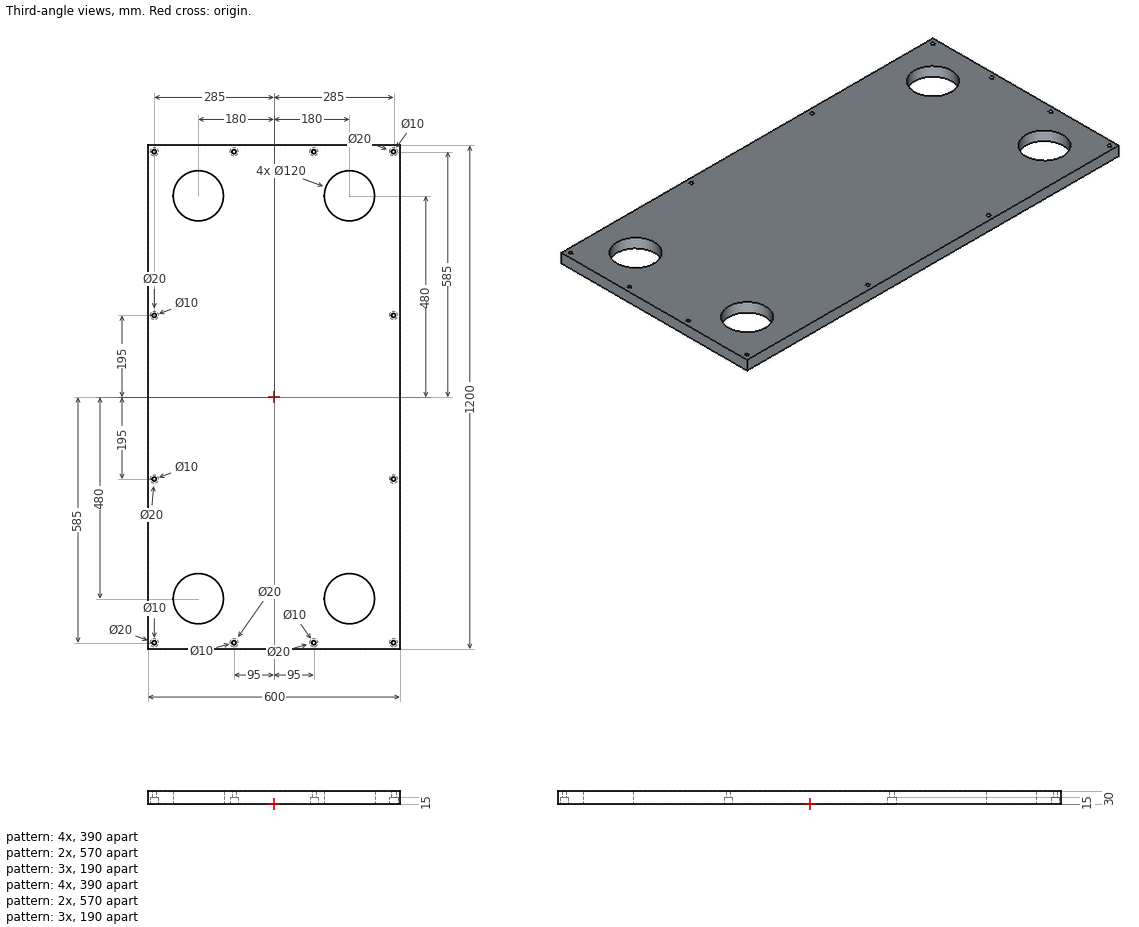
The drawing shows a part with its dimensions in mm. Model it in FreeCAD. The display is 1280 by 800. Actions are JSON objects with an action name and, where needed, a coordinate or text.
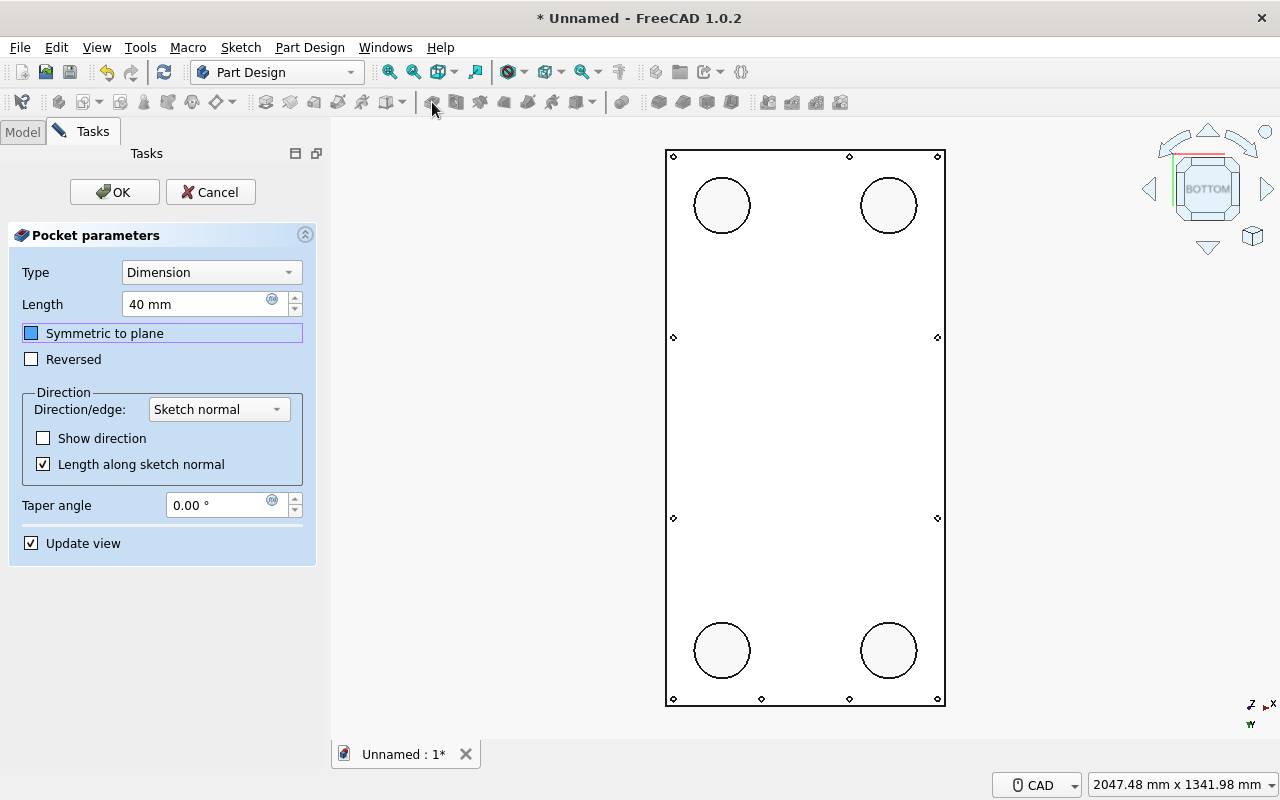
{"action": "left_click", "coordinate": [115, 192]}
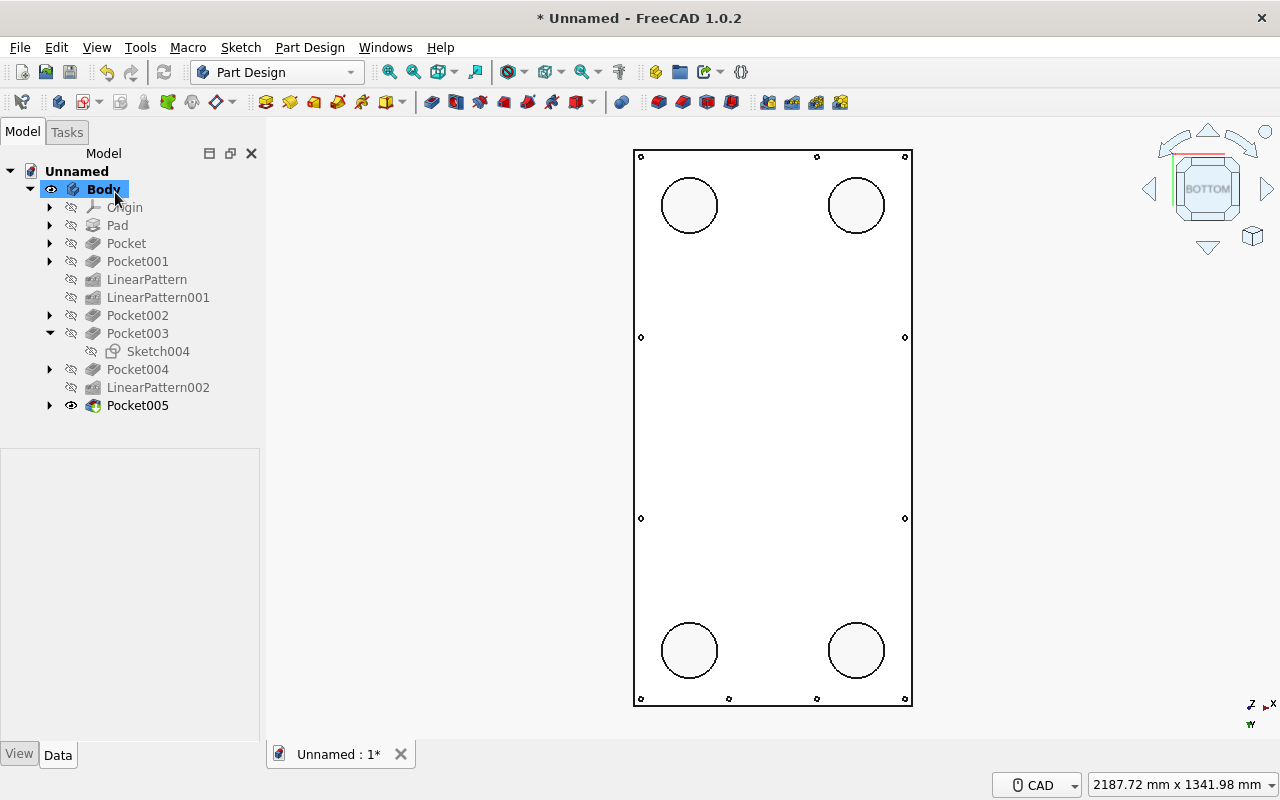
{"action": "left_click", "coordinate": [84, 102]}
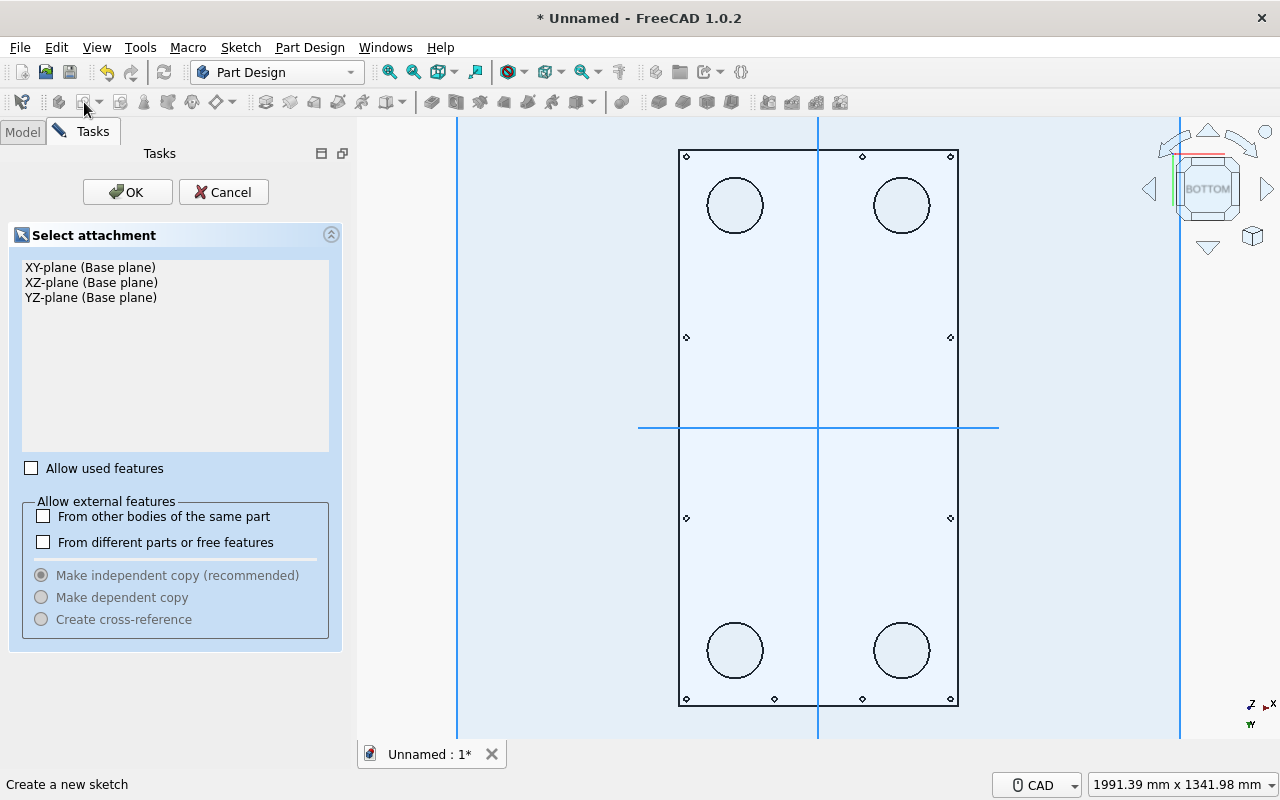
{"action": "left_click", "coordinate": [82, 268]}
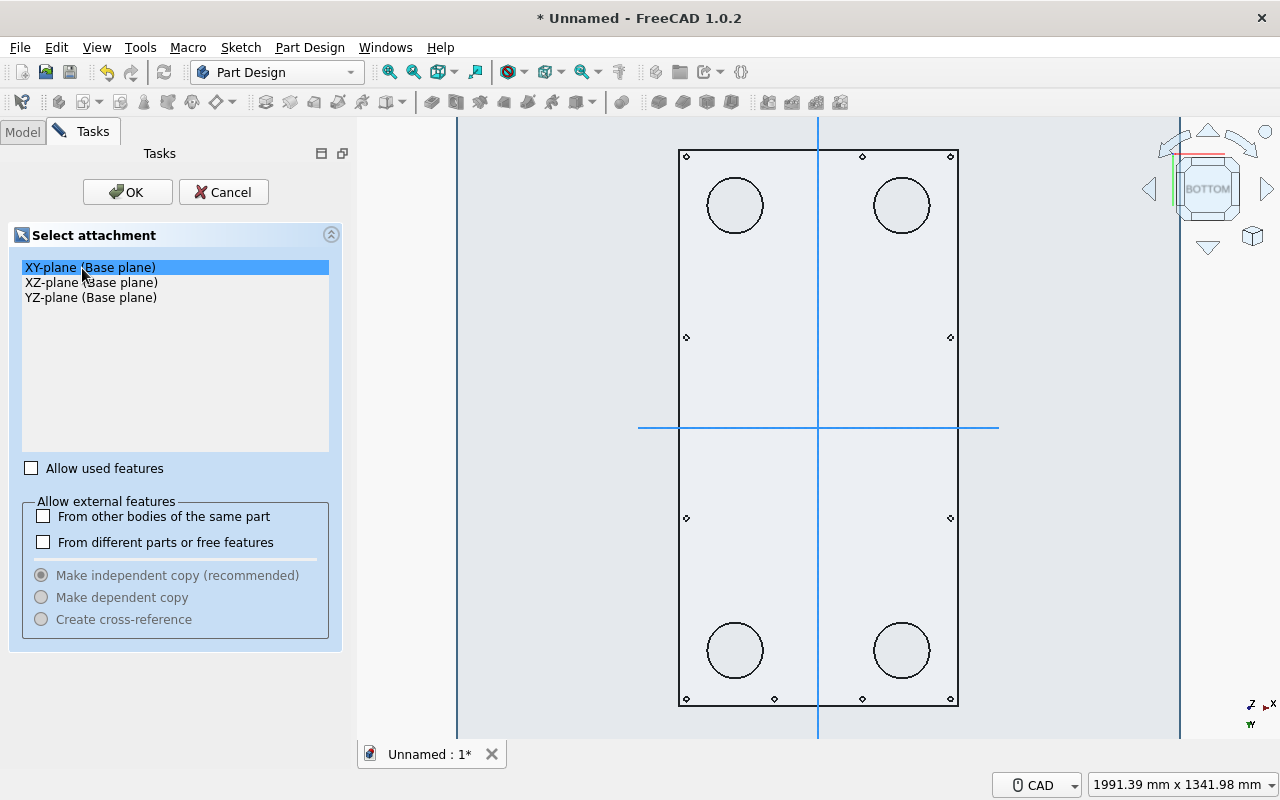
{"action": "left_click", "coordinate": [128, 192]}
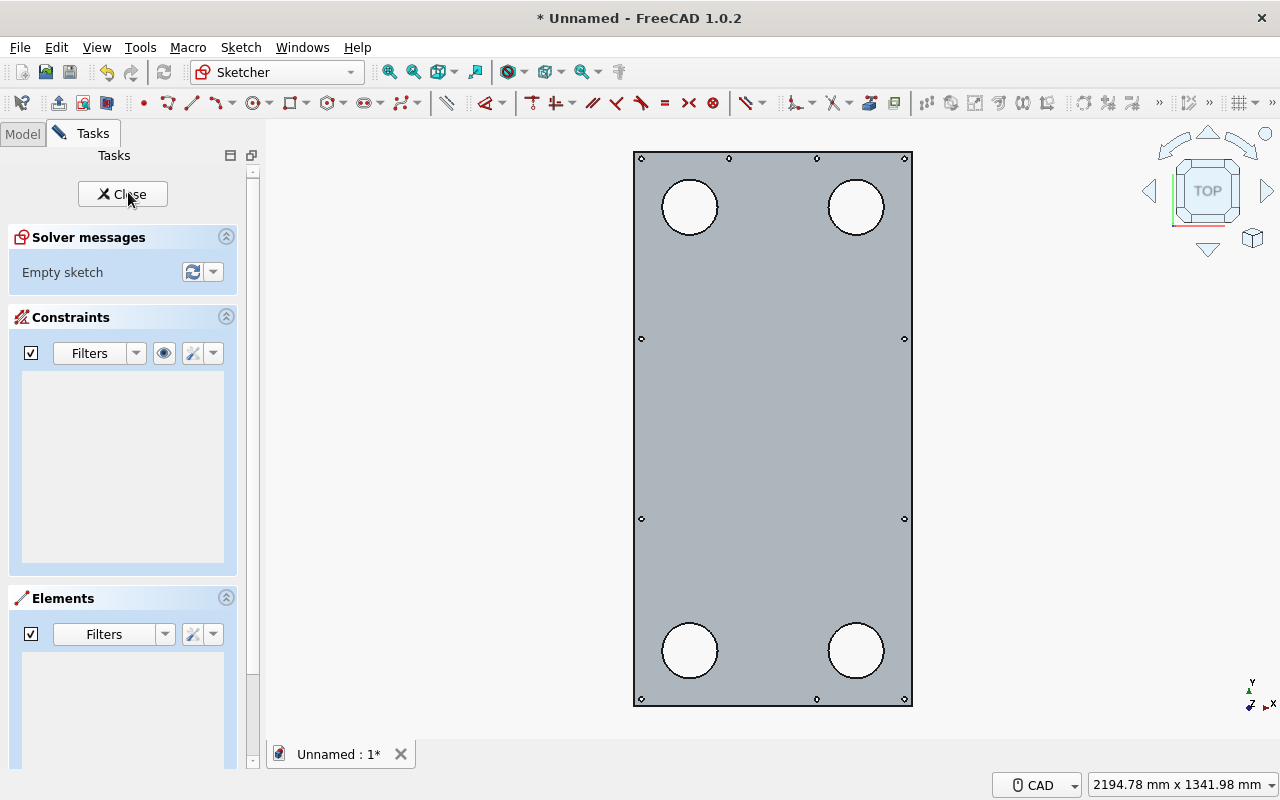
{"action": "left_click", "coordinate": [108, 104]}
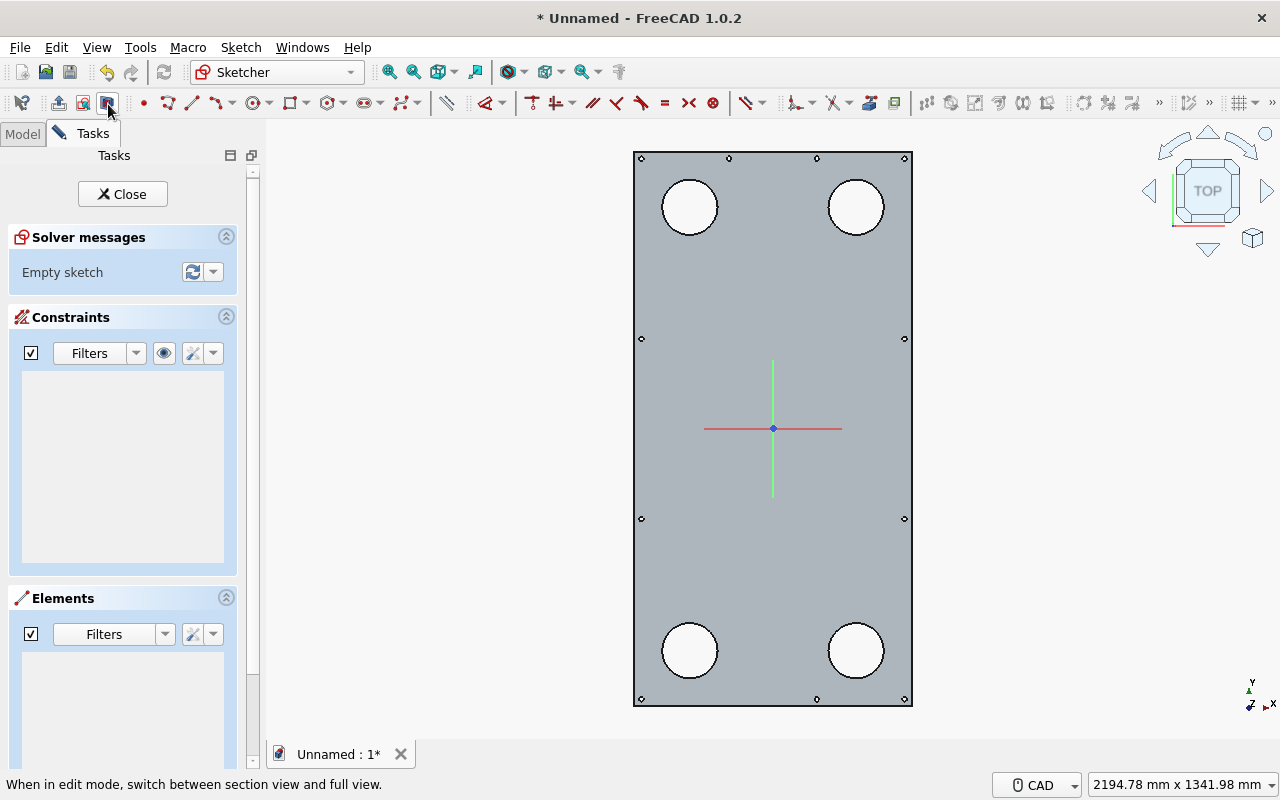
{"action": "scroll", "coordinate": [730, 711], "scroll_direction": "up", "scroll_amount": 15}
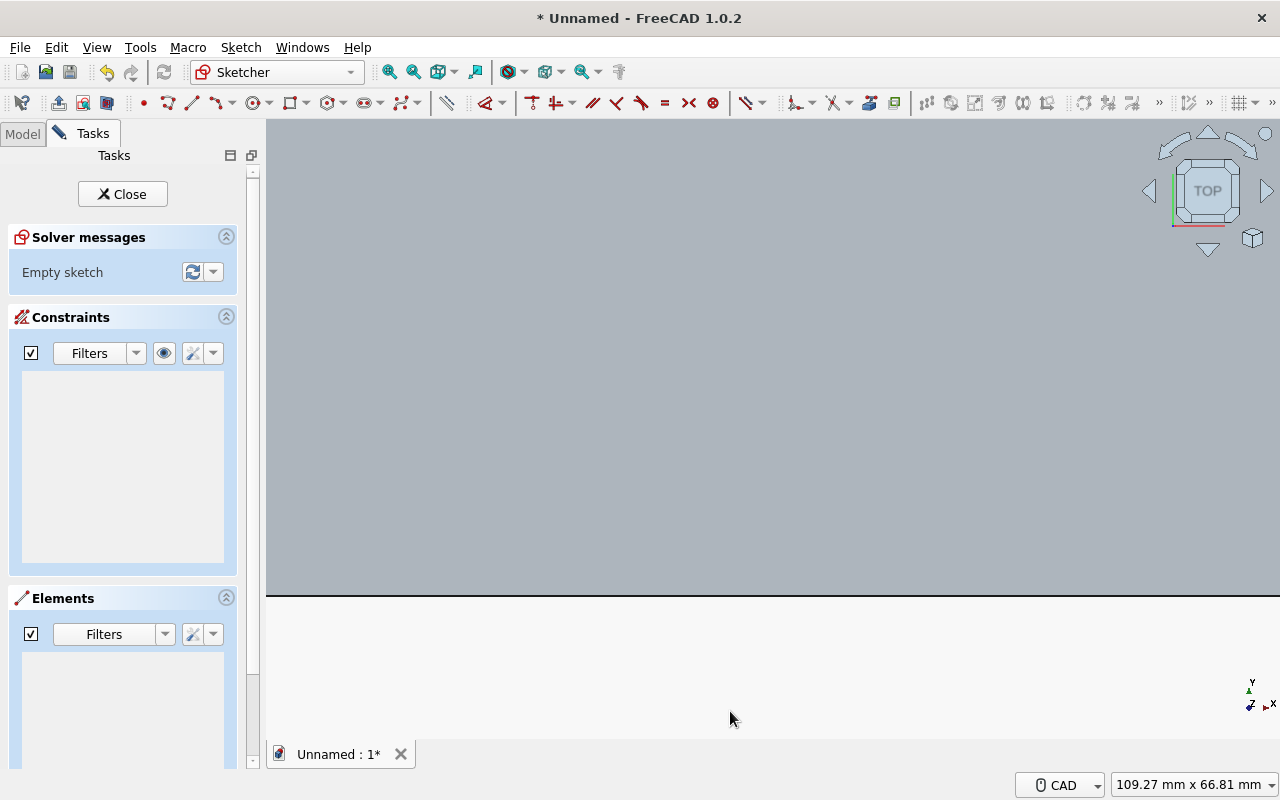
{"action": "scroll", "coordinate": [703, 466], "scroll_direction": "up", "scroll_amount": 7}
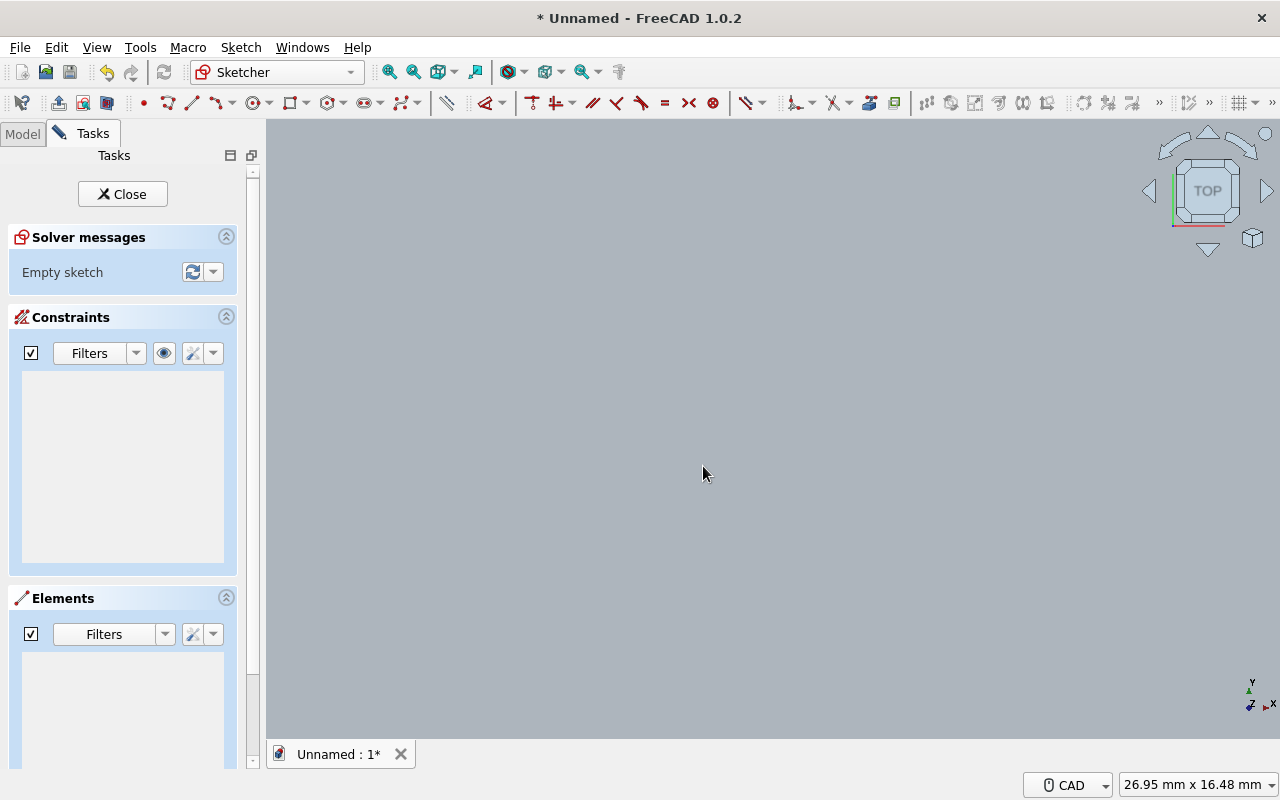
{"action": "left_click", "coordinate": [254, 104]}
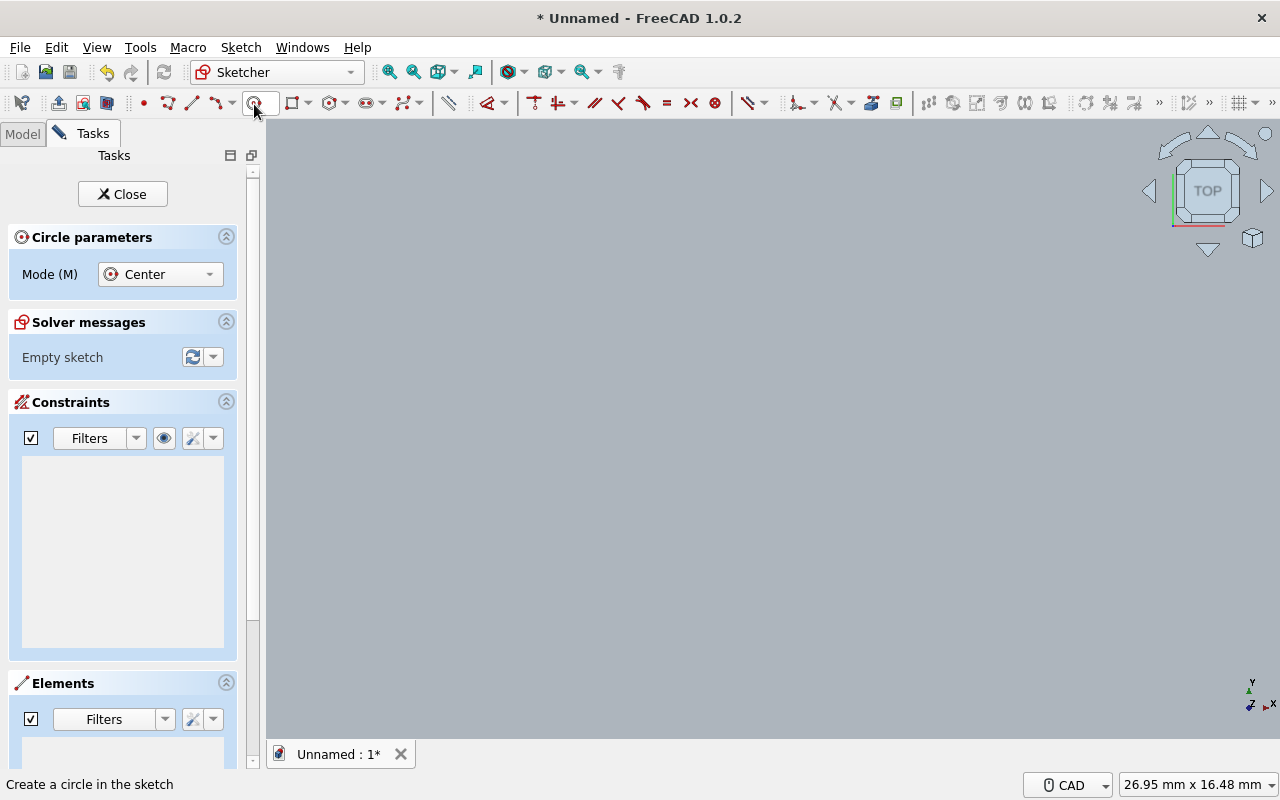
{"action": "left_click", "coordinate": [703, 429]}
{"action": "mouse_move", "coordinate": [836, 296]}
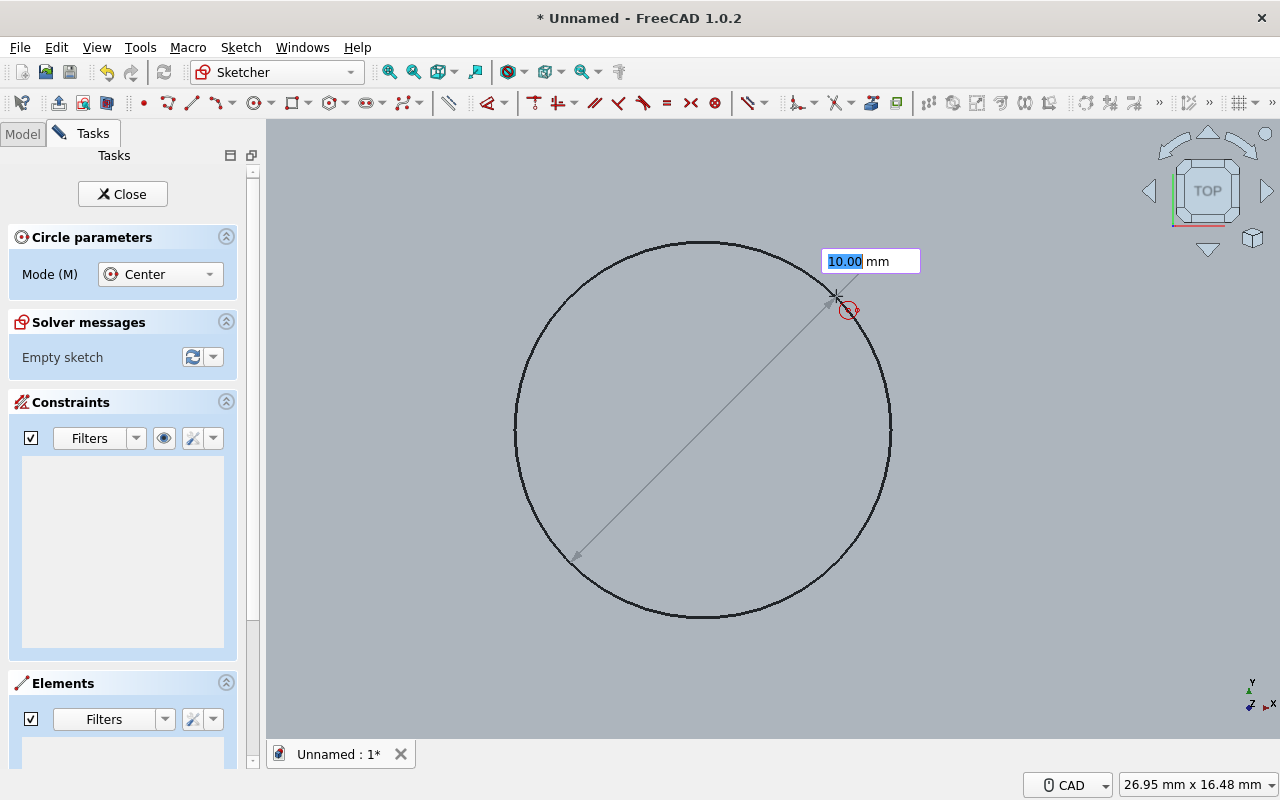
{"action": "type", "text": "10"}
{"action": "key", "text": "Return"}
{"action": "key", "text": "Escape"}